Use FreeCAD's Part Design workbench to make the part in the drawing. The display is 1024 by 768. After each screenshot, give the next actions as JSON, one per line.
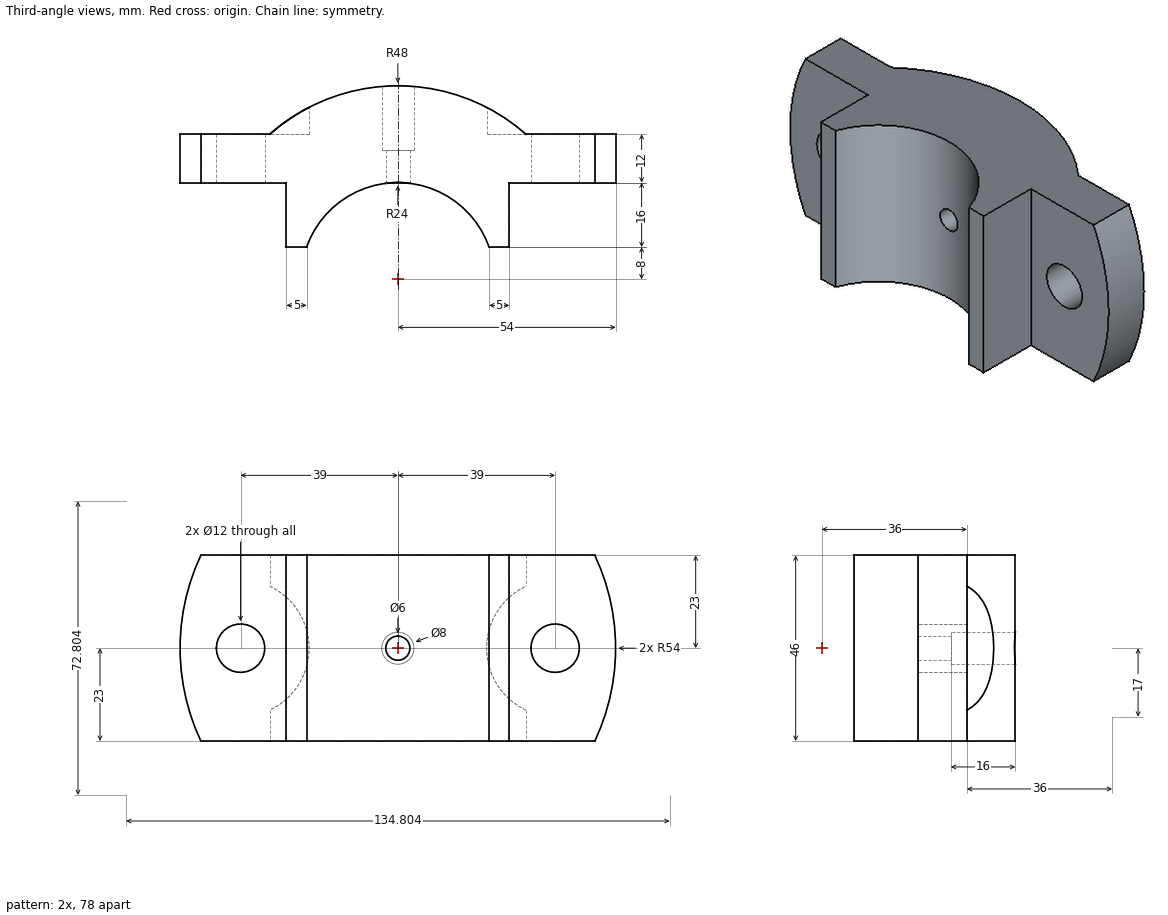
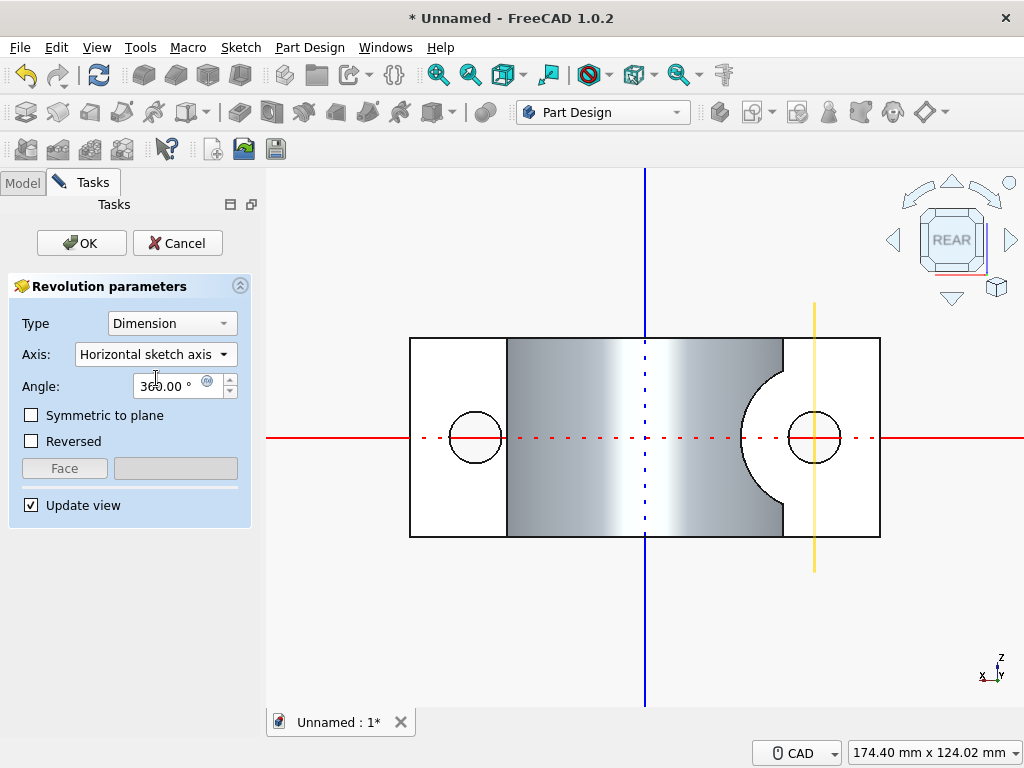
{"action": "left_click", "coordinate": [82, 243]}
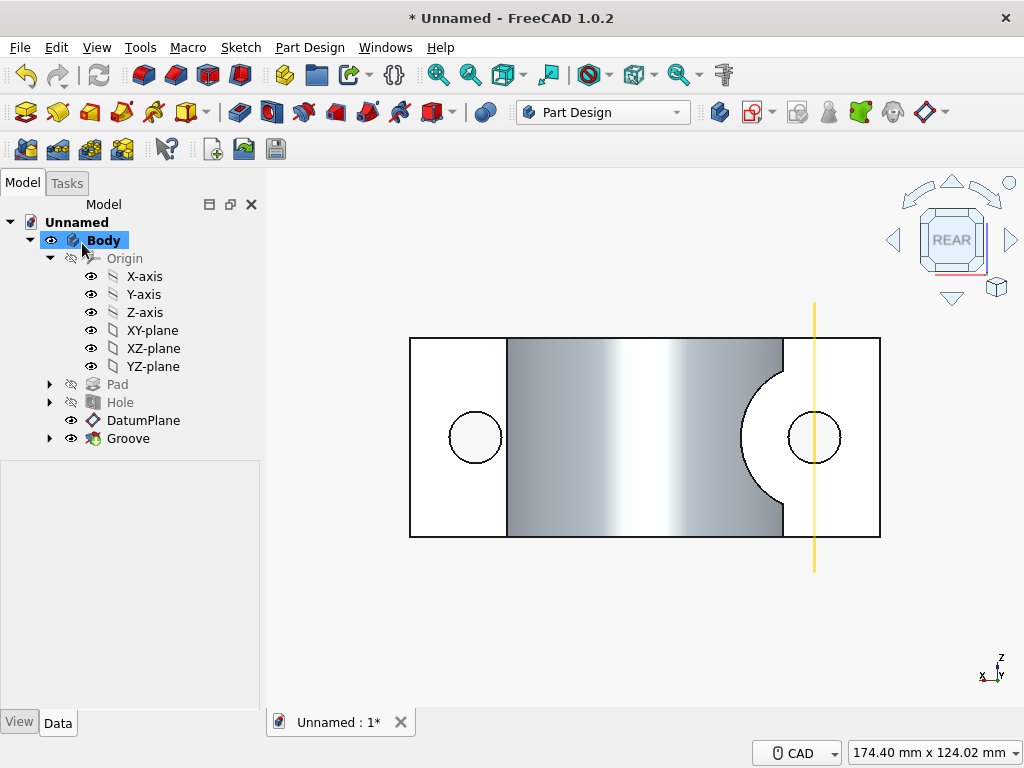
{"action": "left_click", "coordinate": [116, 420]}
{"action": "key", "text": "space"}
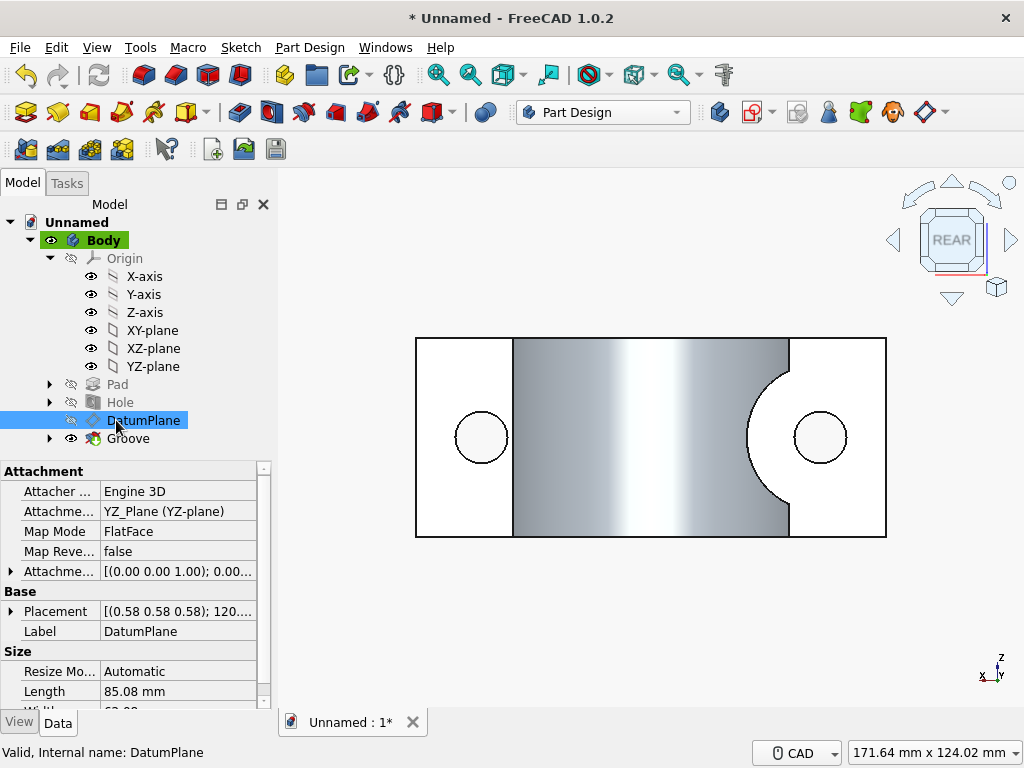
{"action": "left_click", "coordinate": [116, 438]}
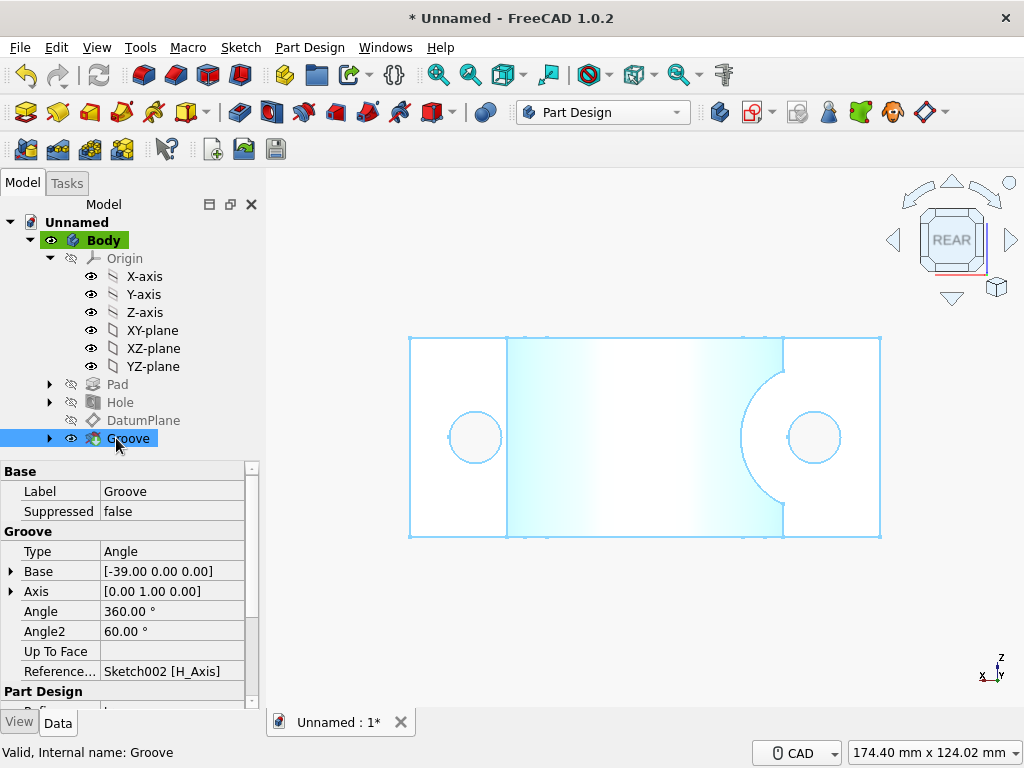
{"action": "left_click", "coordinate": [58, 150]}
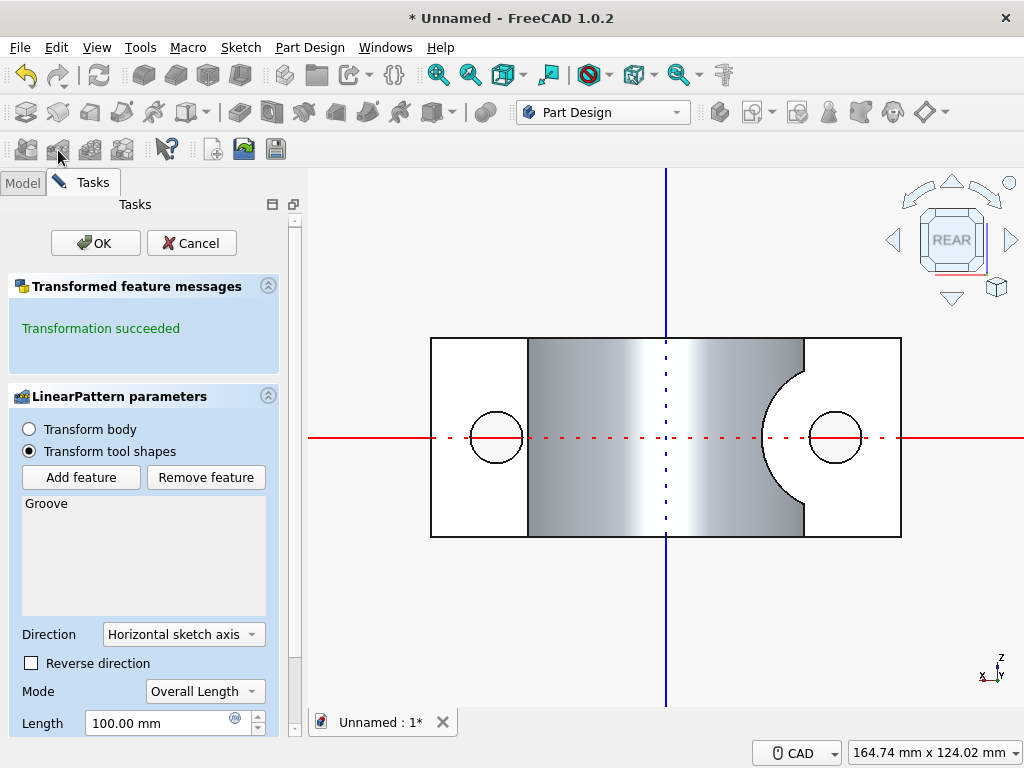
{"action": "left_click", "coordinate": [184, 634]}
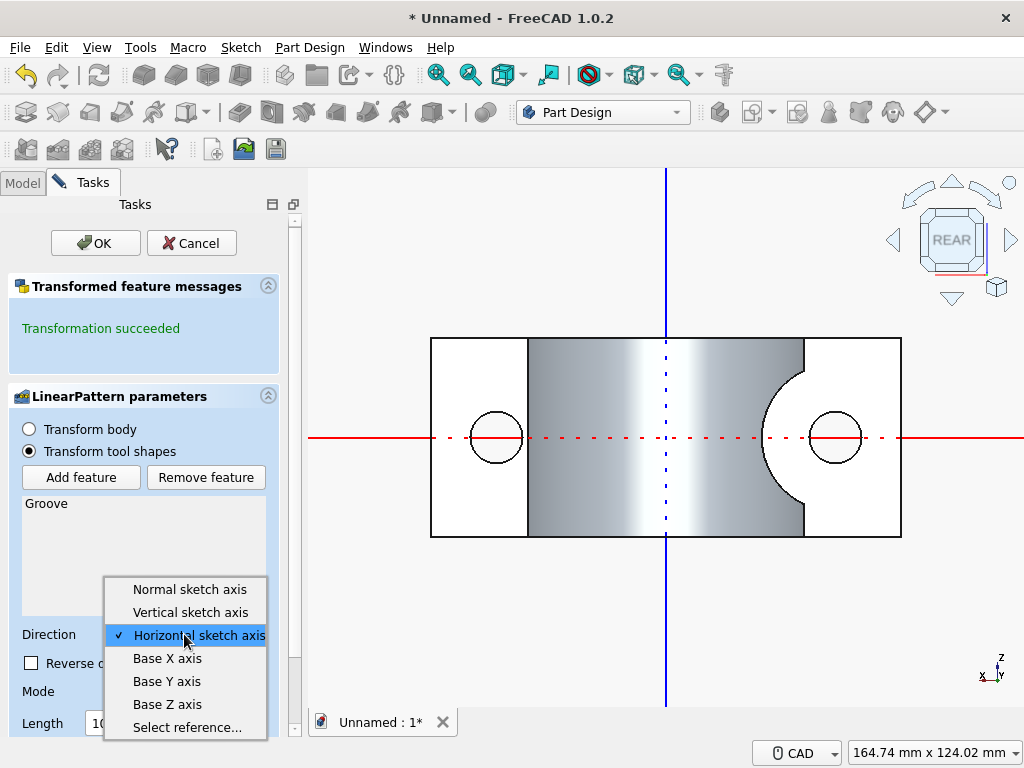
{"action": "left_click", "coordinate": [184, 658]}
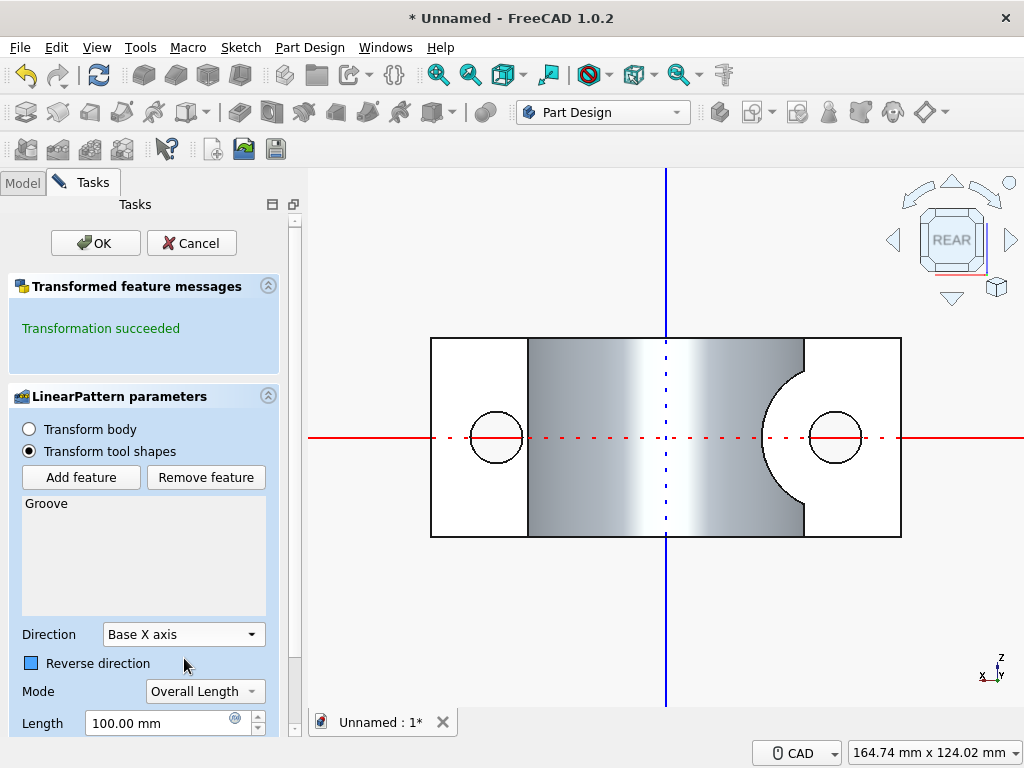
{"action": "left_click", "coordinate": [206, 692]}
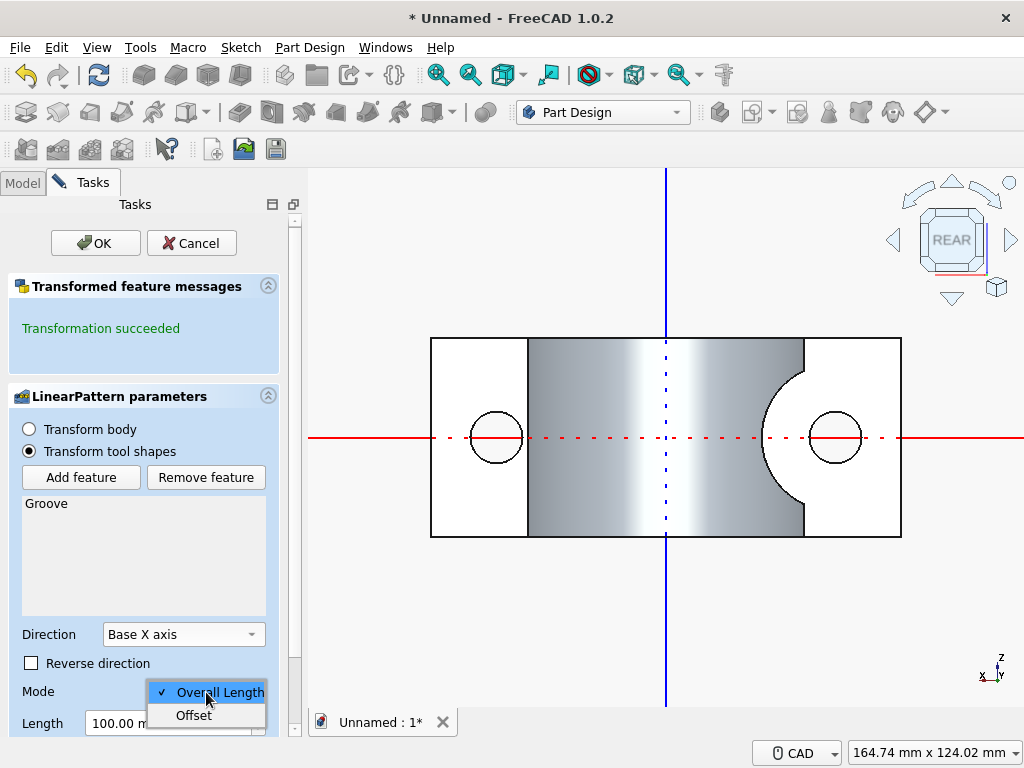
{"action": "left_click", "coordinate": [206, 716]}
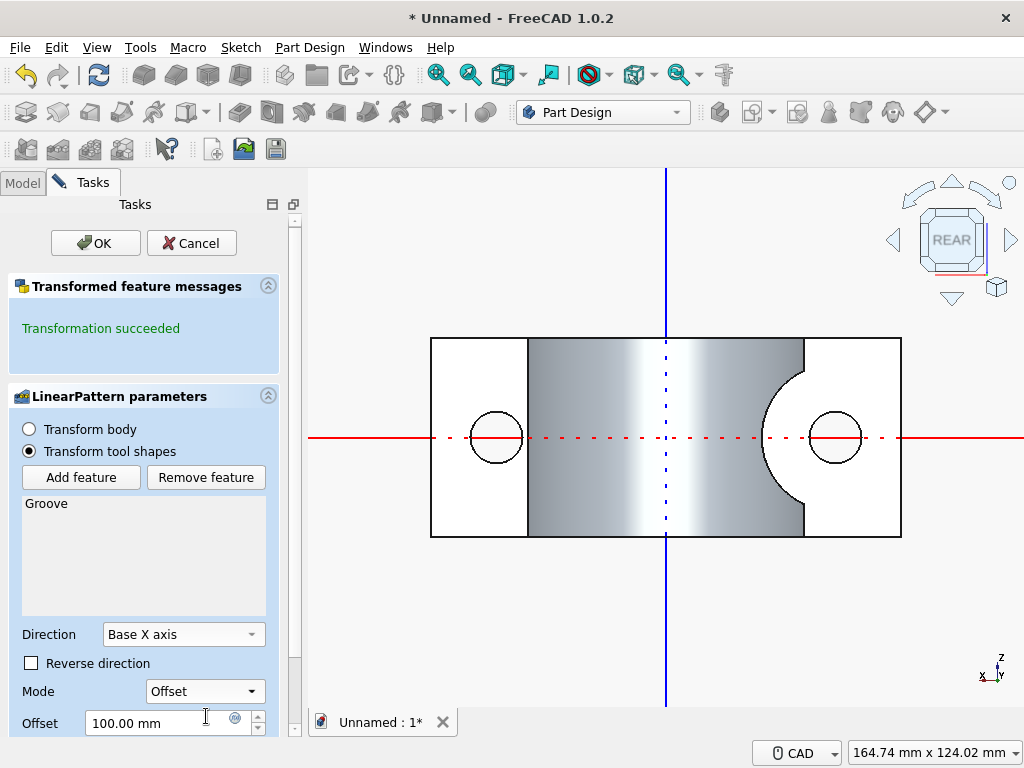
{"action": "triple_click", "coordinate": [168, 723]}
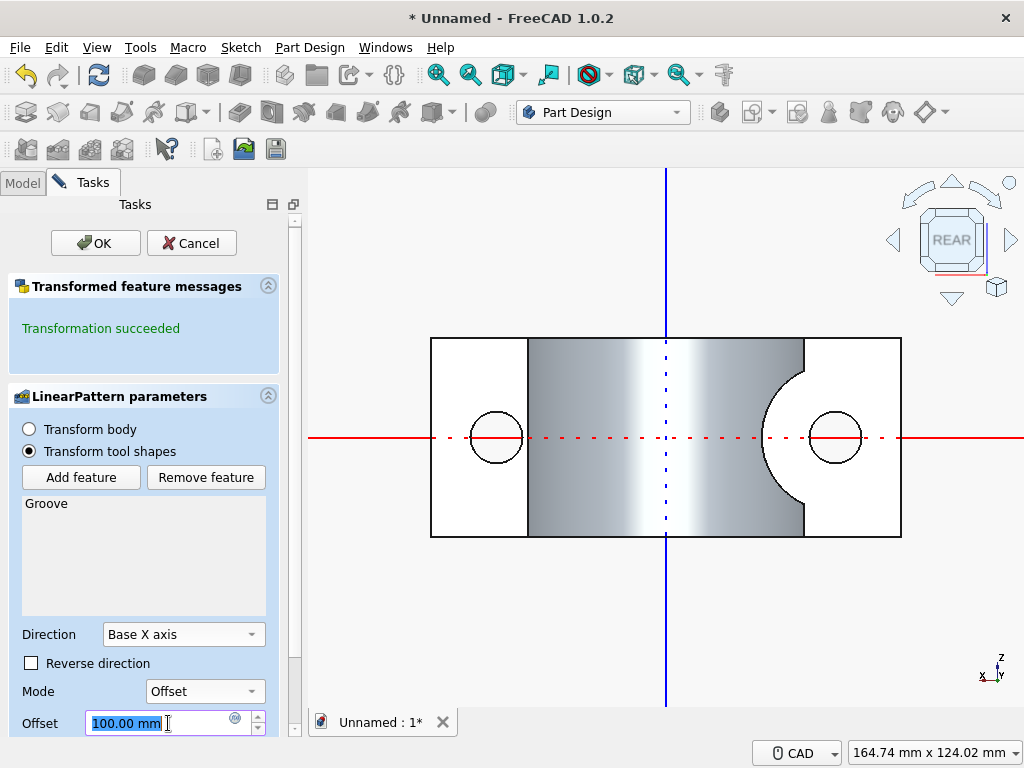
{"action": "type", "text": "78"}
{"action": "key", "text": "Tab"}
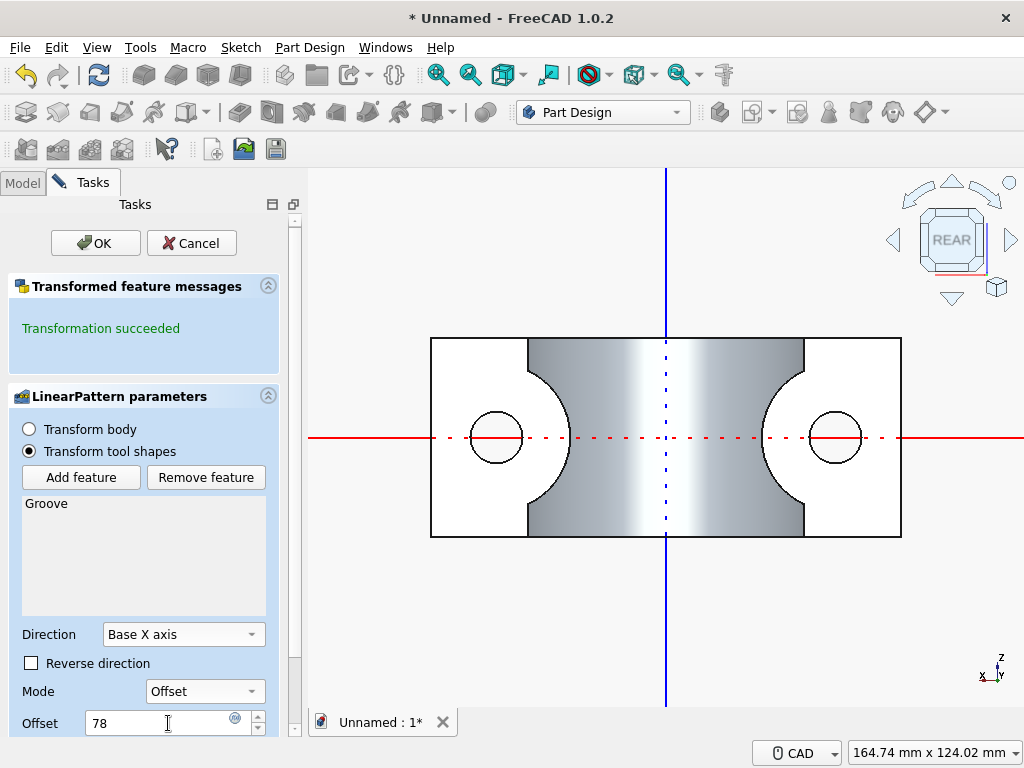
{"action": "scroll", "coordinate": [295, 475], "scroll_direction": "down", "scroll_amount": 2}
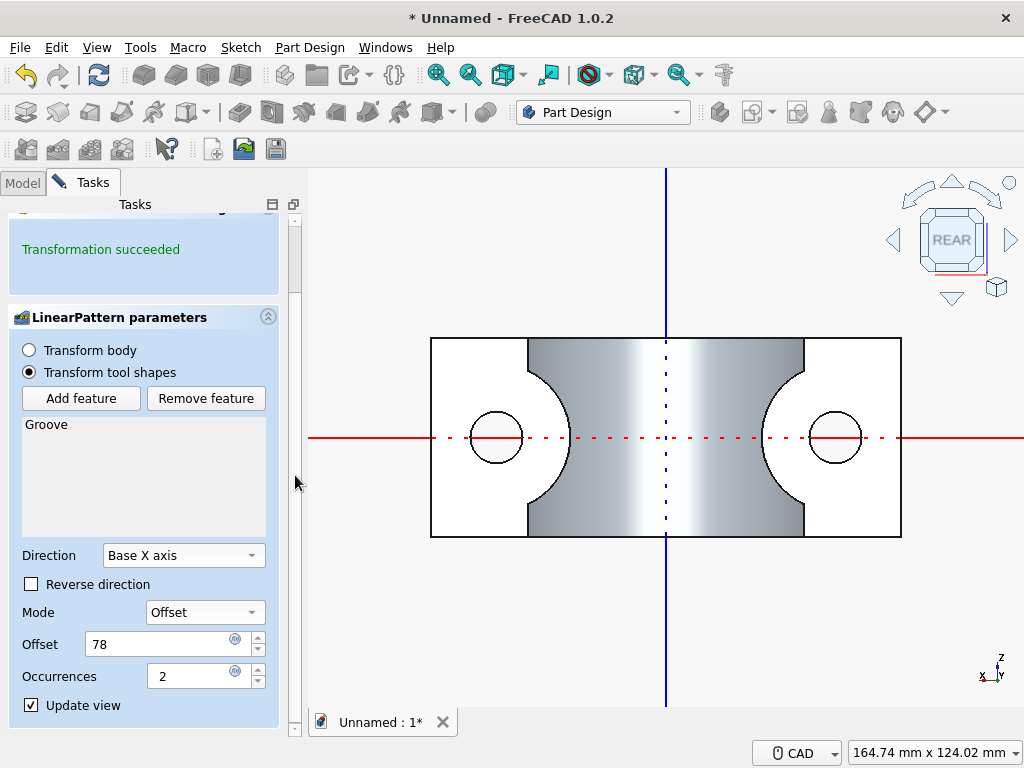
{"action": "triple_click", "coordinate": [198, 676]}